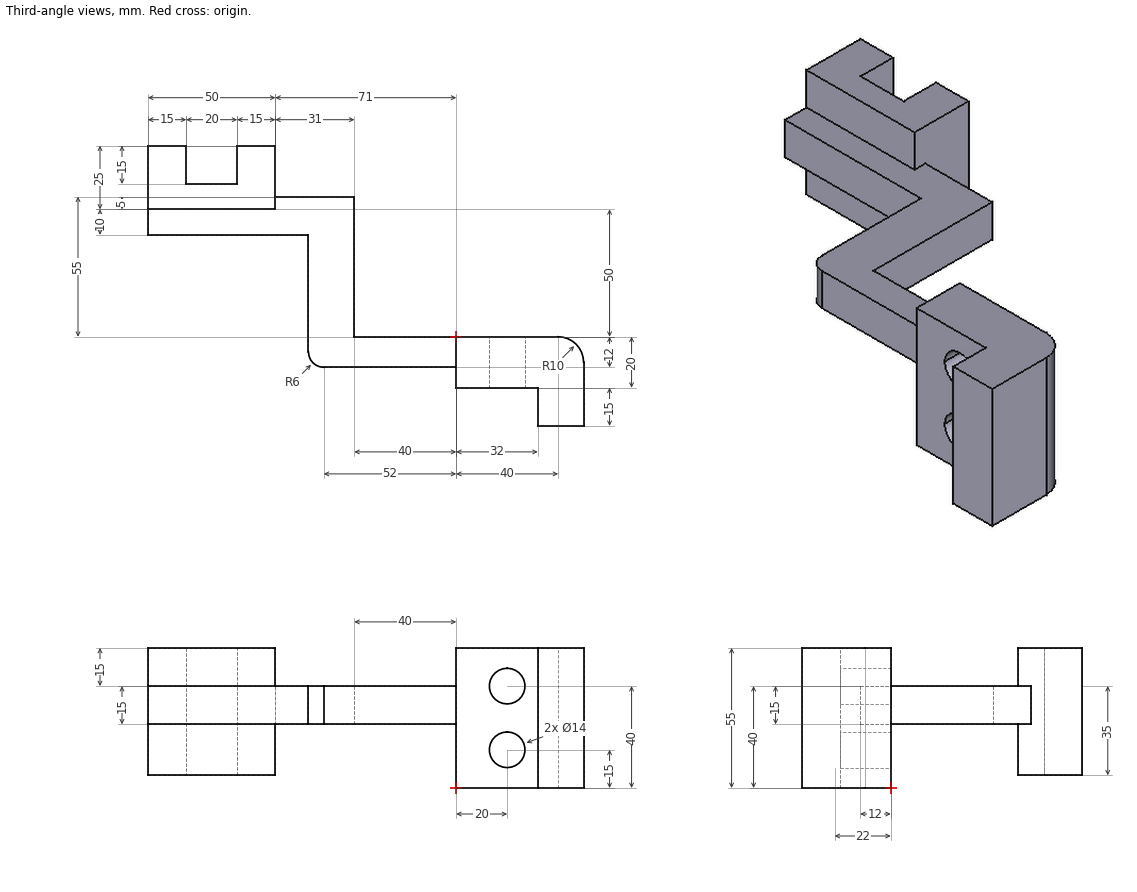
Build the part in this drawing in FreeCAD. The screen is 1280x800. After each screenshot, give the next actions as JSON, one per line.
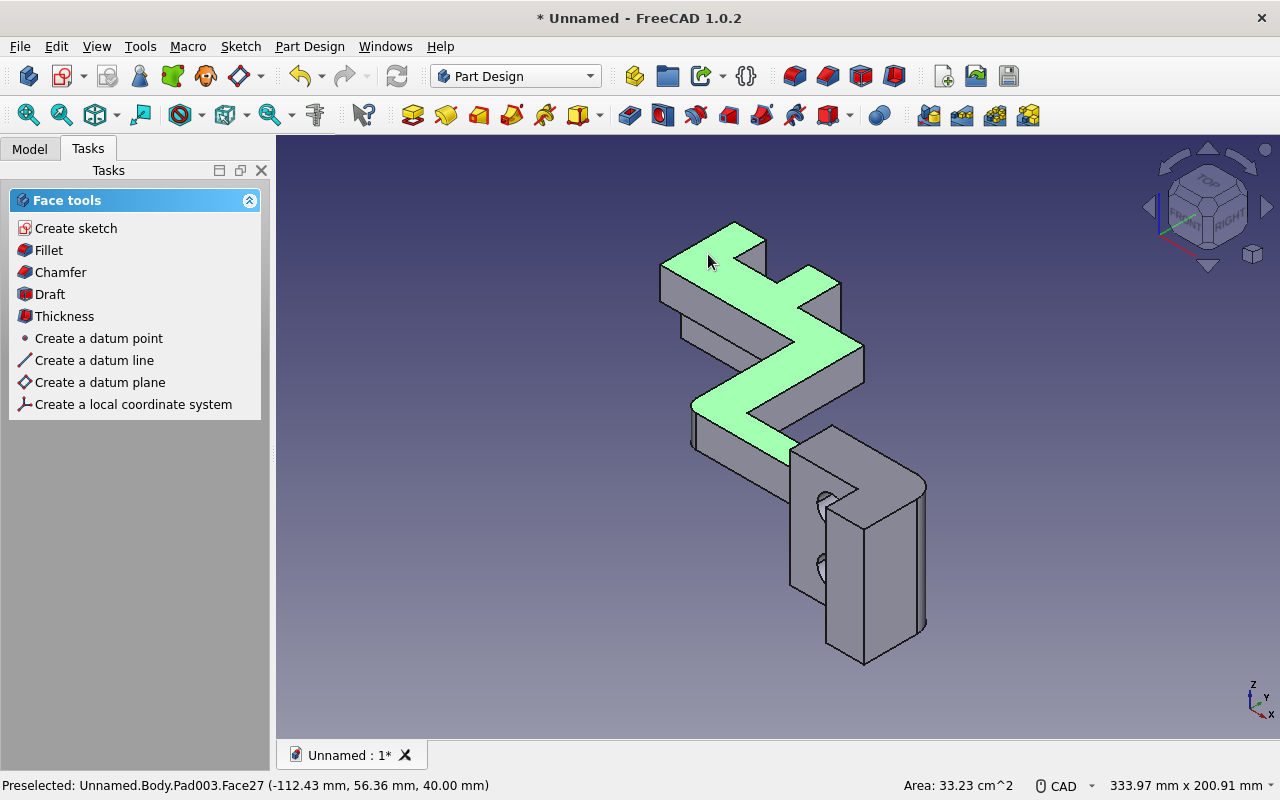
{"action": "left_click", "coordinate": [62, 76]}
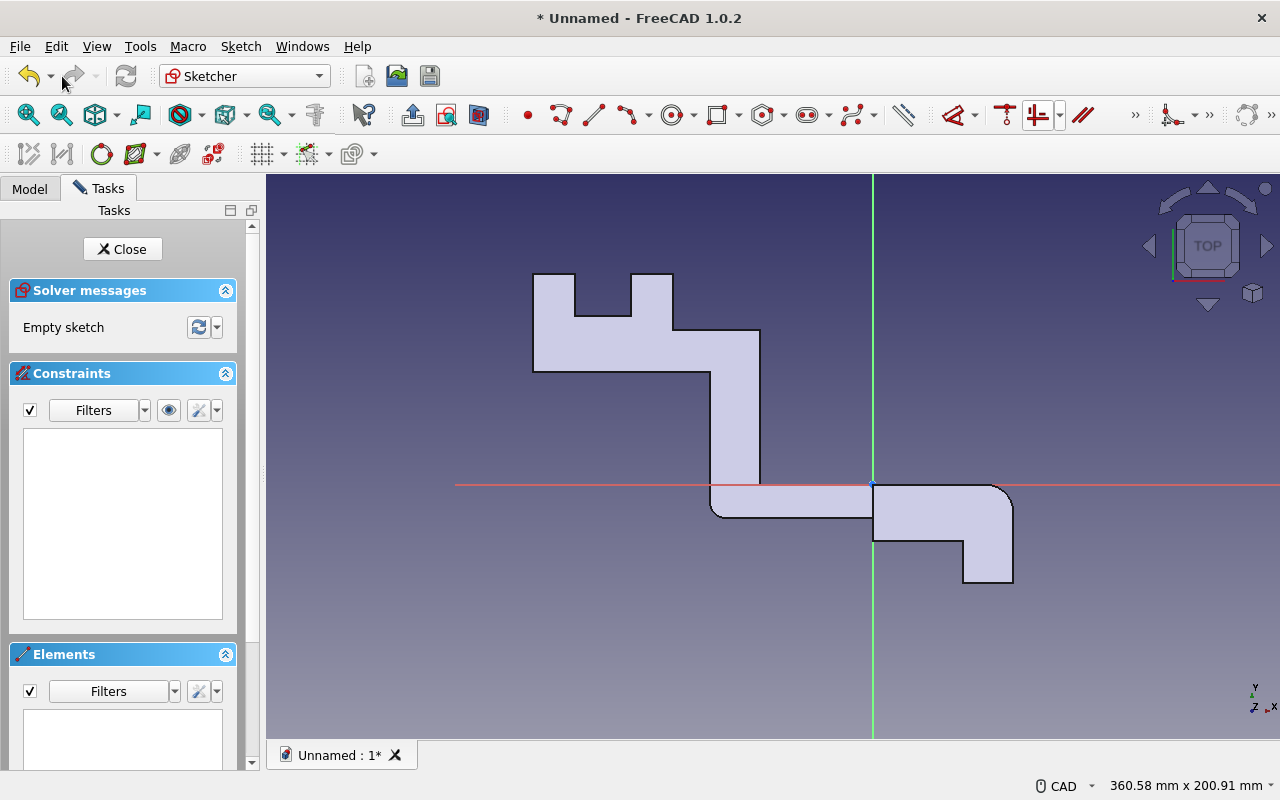
{"action": "scroll", "coordinate": [701, 285], "scroll_direction": "up", "scroll_amount": 3}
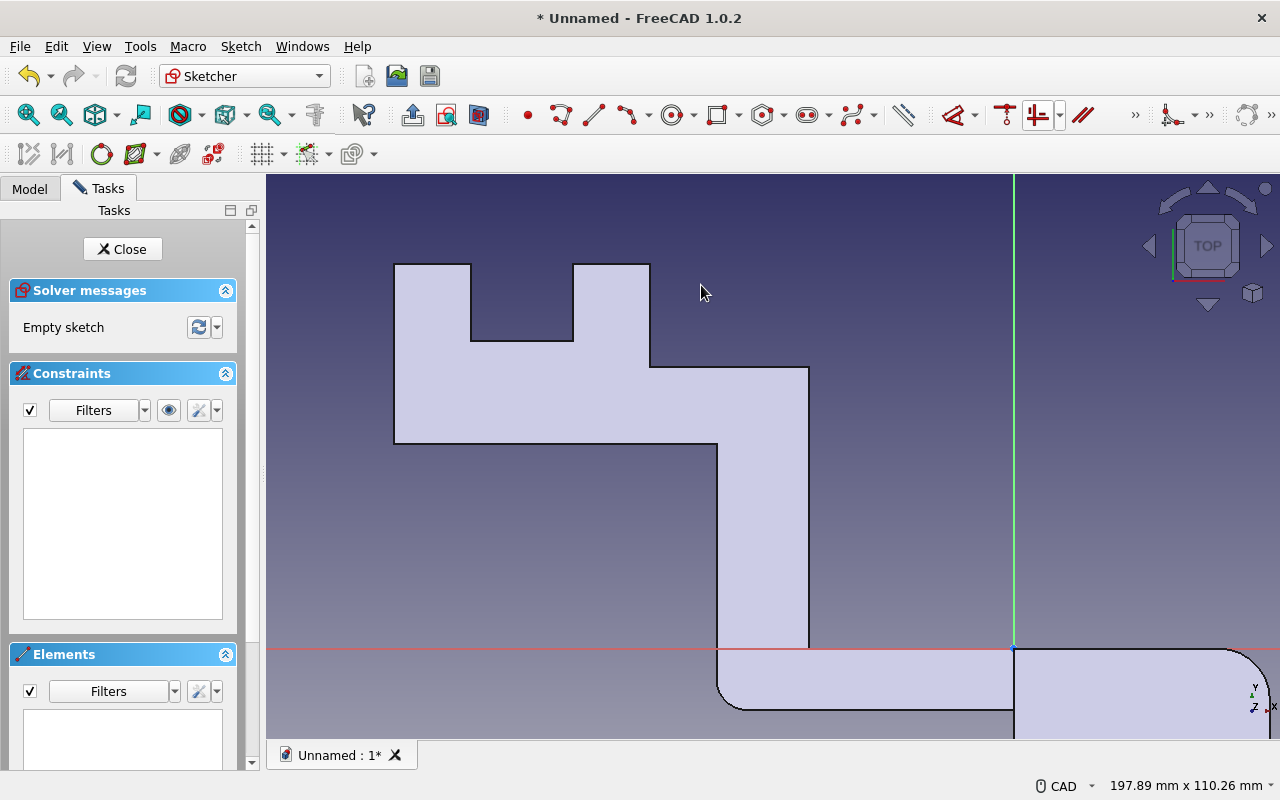
{"action": "left_click", "coordinate": [561, 116]}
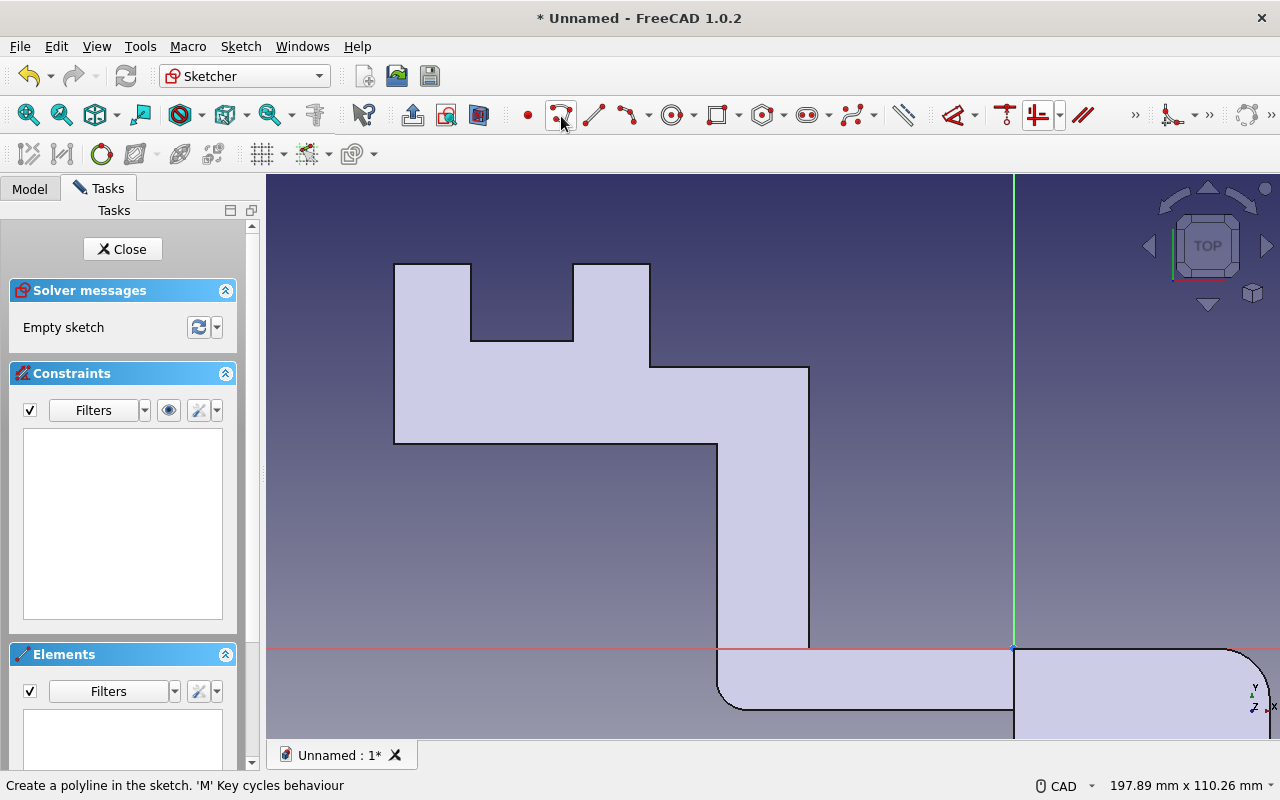
{"action": "left_click", "coordinate": [650, 392]}
{"action": "left_click", "coordinate": [650, 264]}
{"action": "left_click", "coordinate": [573, 264]}
{"action": "left_click", "coordinate": [573, 341]}
{"action": "left_click", "coordinate": [471, 341]}
{"action": "left_click", "coordinate": [471, 264]}
{"action": "left_click", "coordinate": [394, 264]}
{"action": "left_click", "coordinate": [394, 392]}
{"action": "left_click", "coordinate": [650, 393]}
{"action": "key", "text": "Escape"}
{"action": "key", "text": "Escape"}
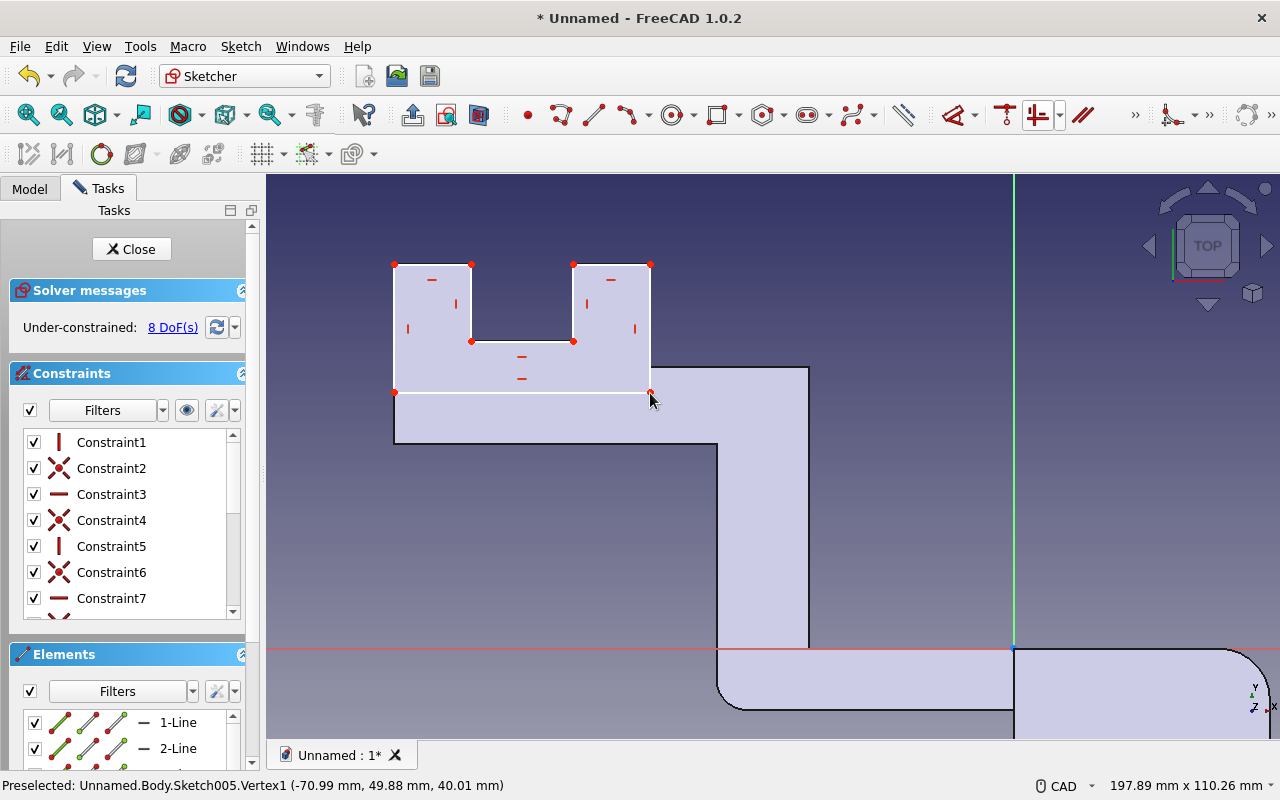
{"action": "left_click", "coordinate": [952, 116]}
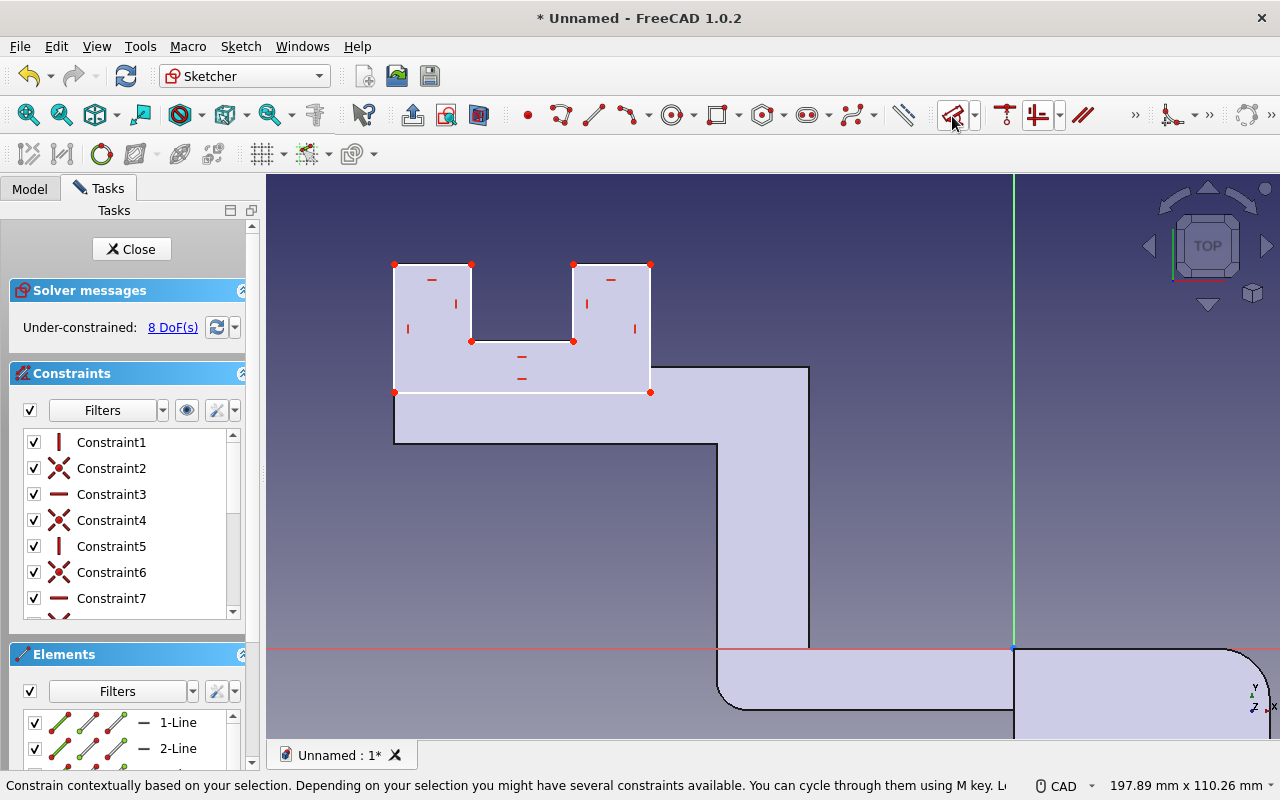
{"action": "left_click", "coordinate": [650, 355]}
{"action": "left_click", "coordinate": [616, 329]}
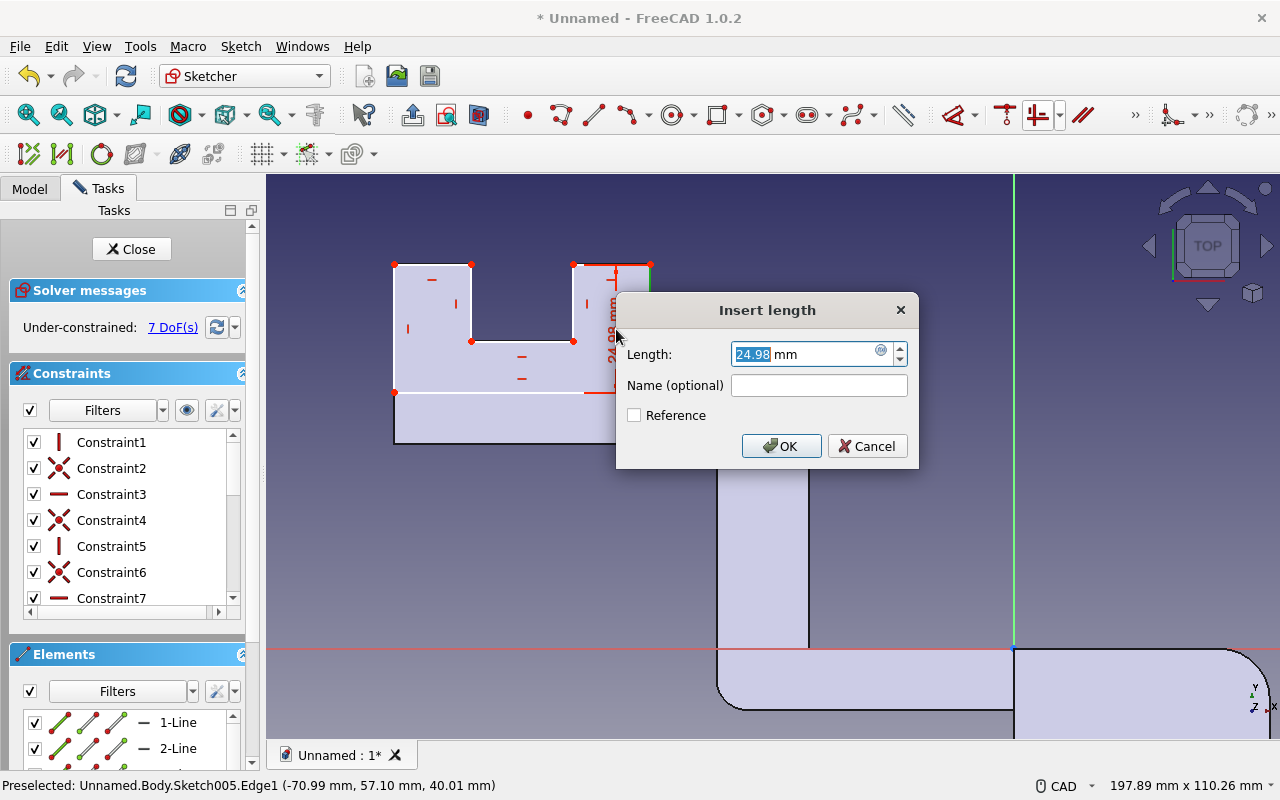
{"action": "type", "text": "25"}
{"action": "key", "text": "Return"}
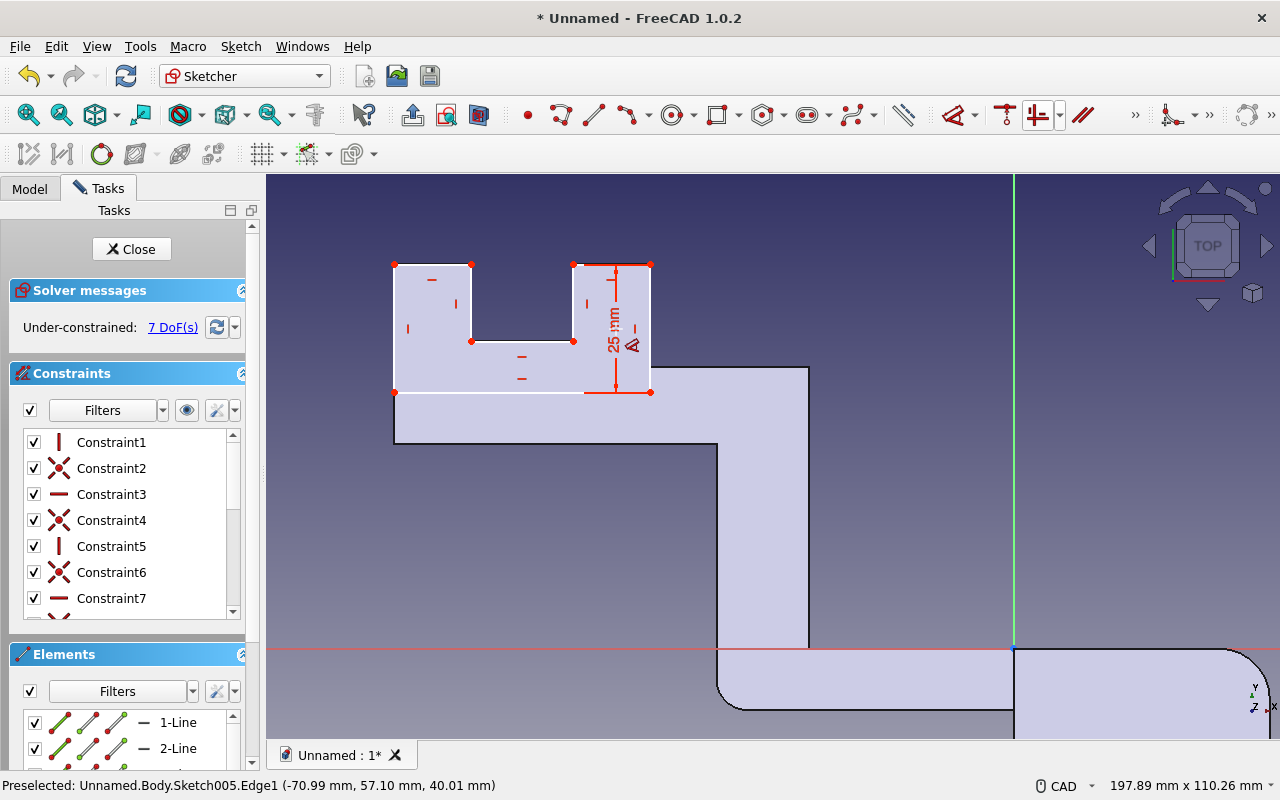
{"action": "left_click", "coordinate": [627, 265]}
{"action": "left_click", "coordinate": [611, 231]}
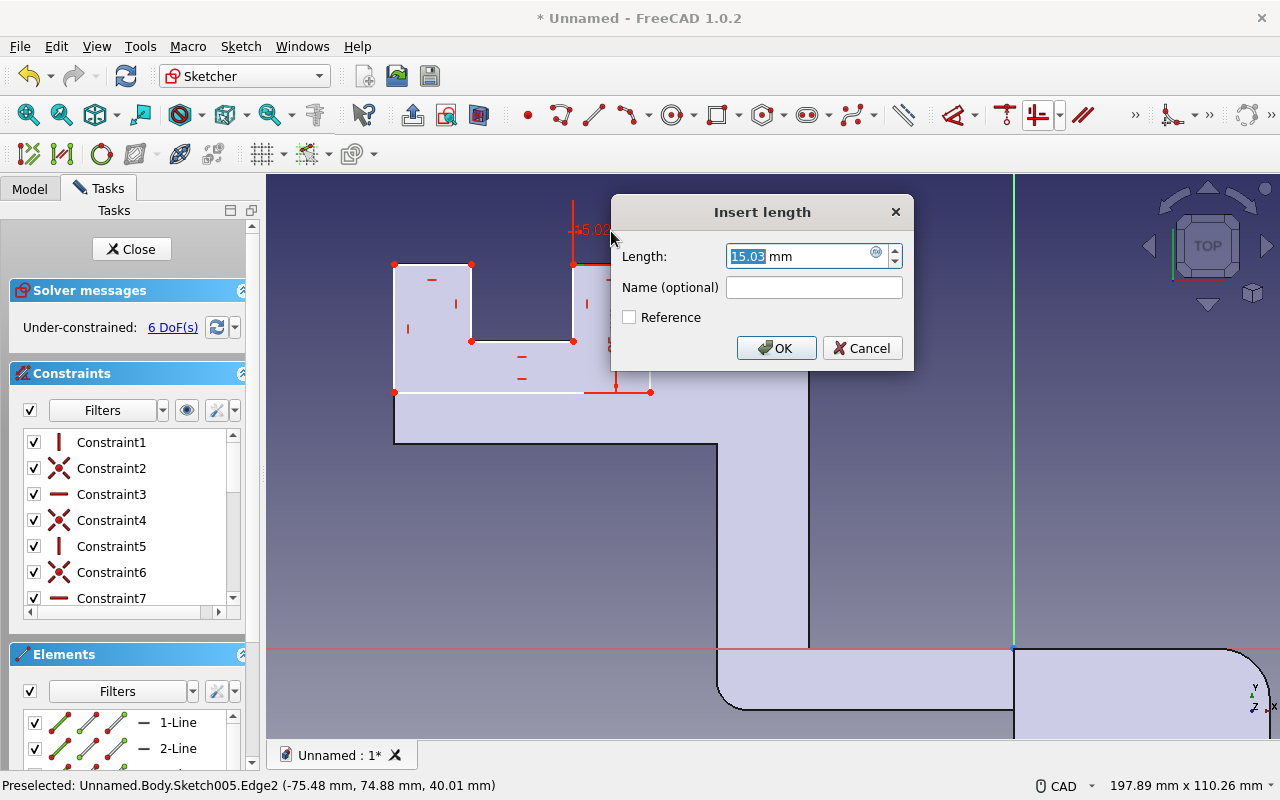
{"action": "type", "text": "15"}
{"action": "key", "text": "Return"}